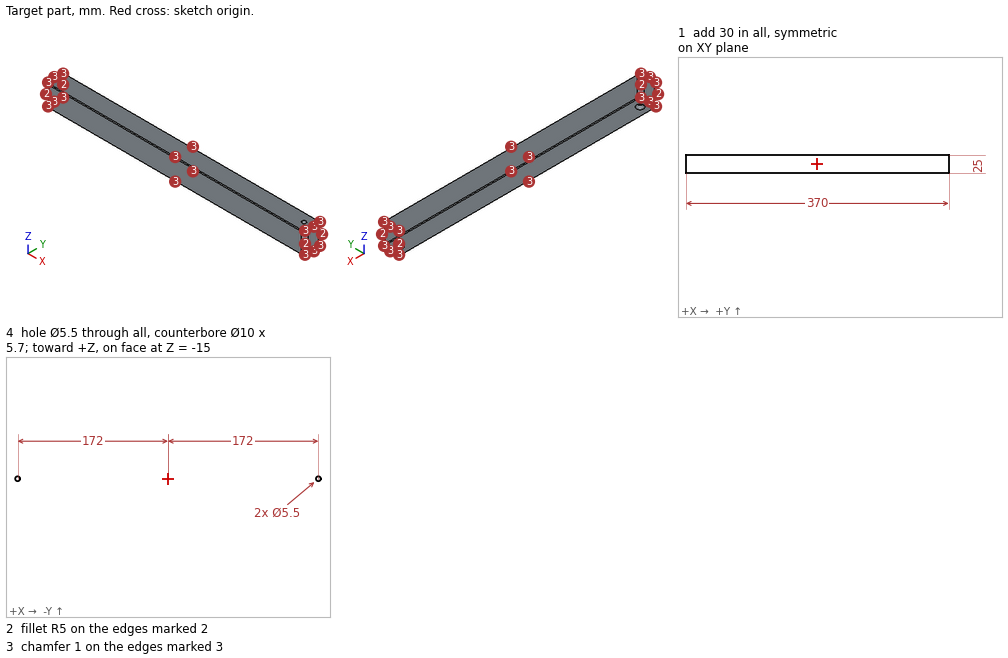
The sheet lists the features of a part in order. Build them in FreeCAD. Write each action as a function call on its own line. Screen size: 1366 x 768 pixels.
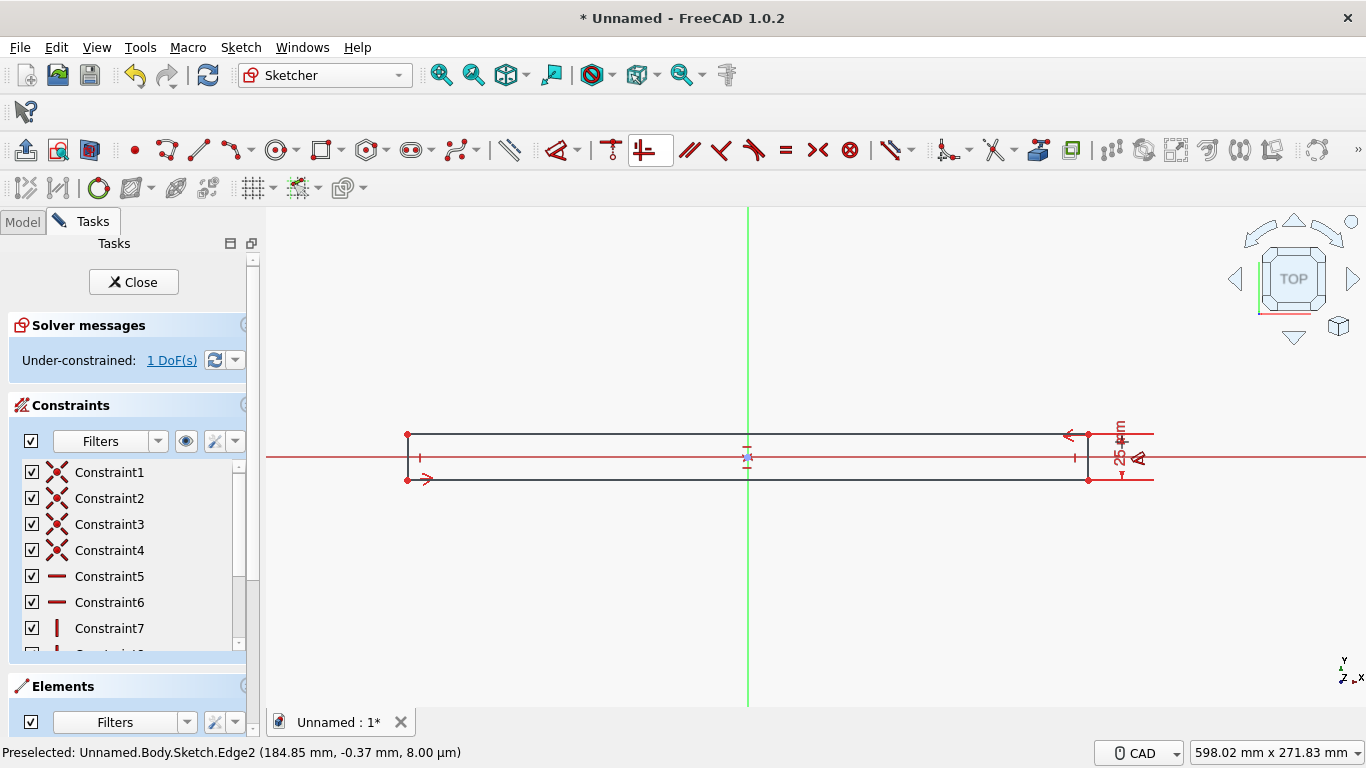
click(612, 480)
click(592, 514)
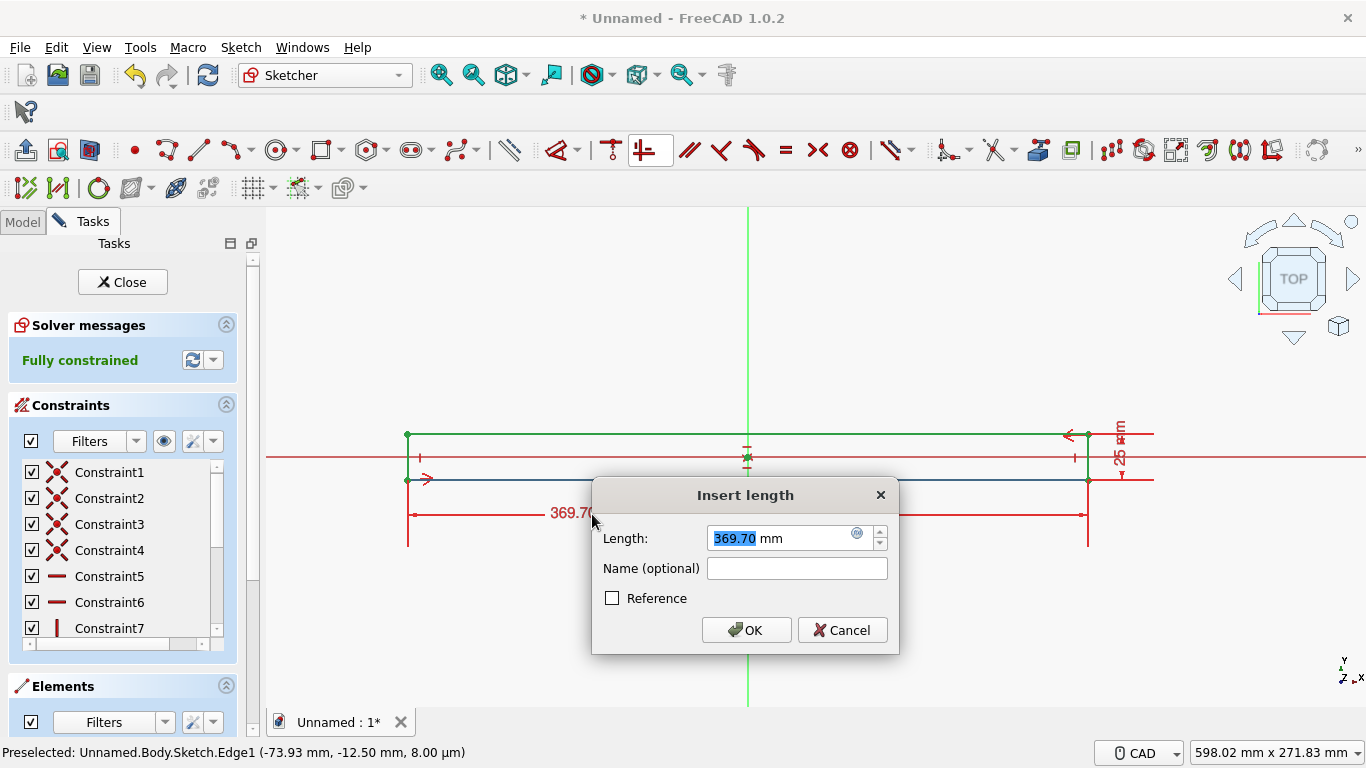
text(370)
key(Return)
key(Escape)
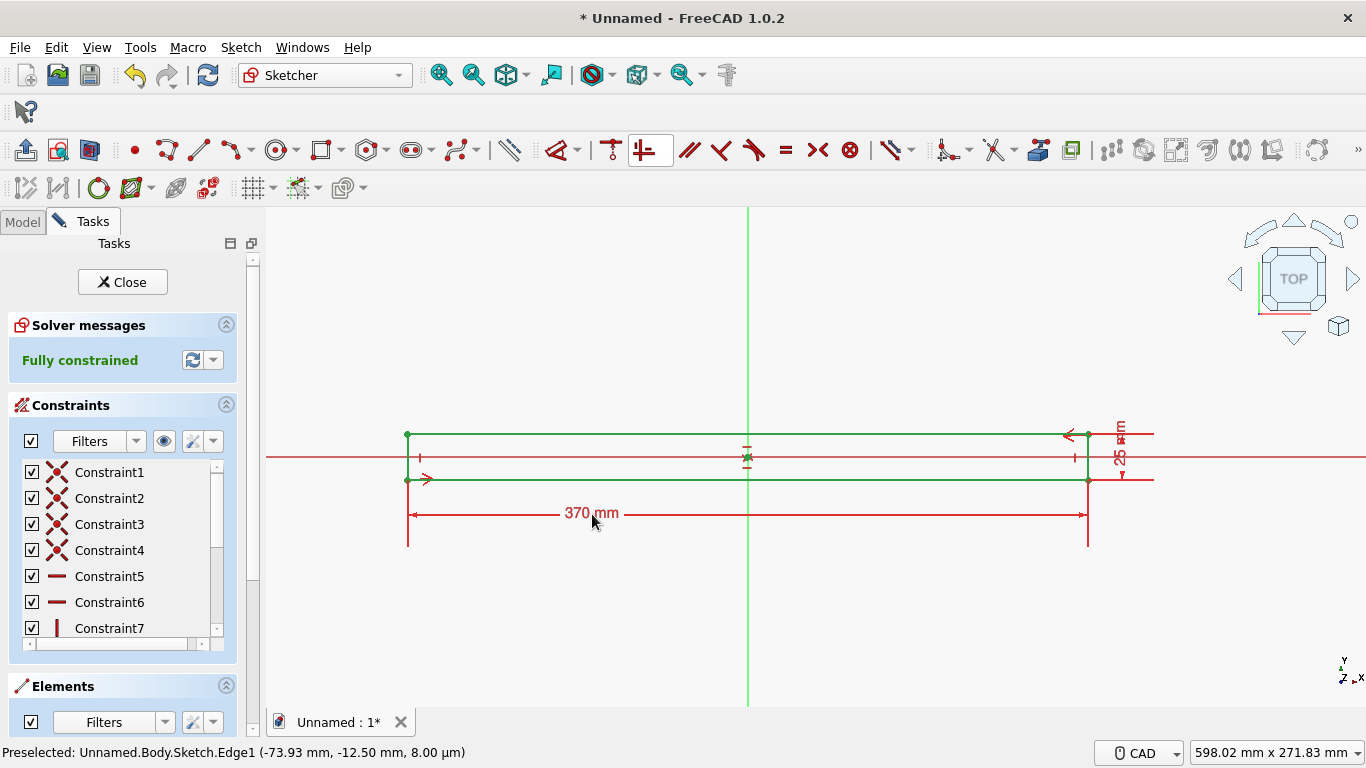
click(123, 282)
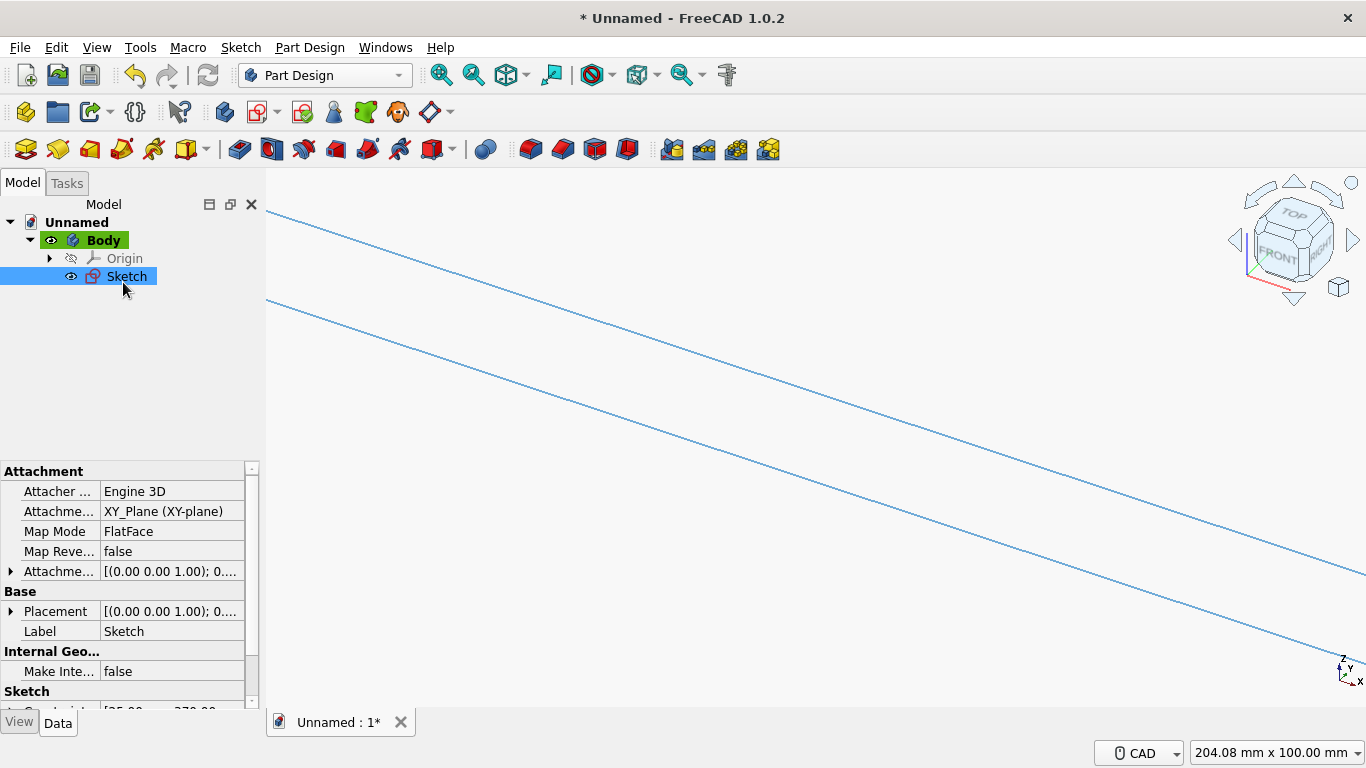
click(26, 150)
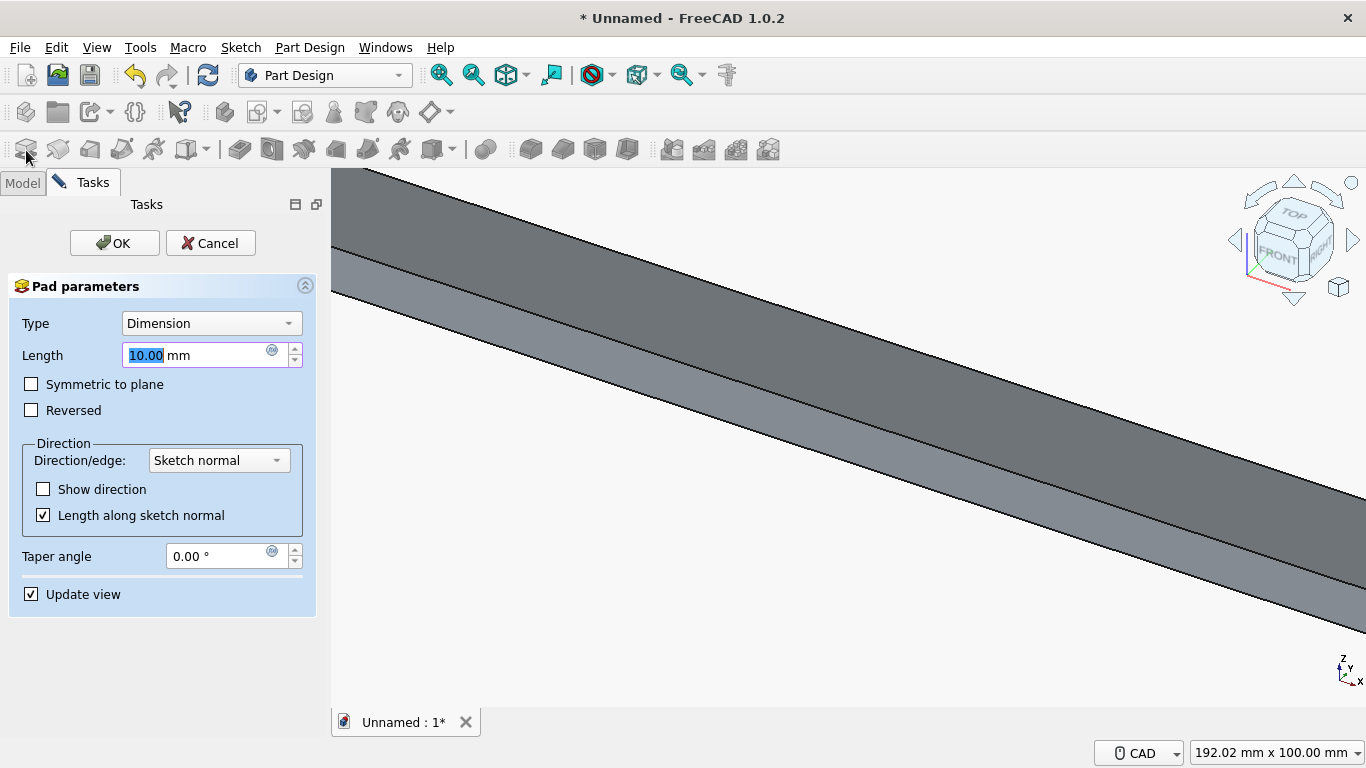
text(30)
key(Tab)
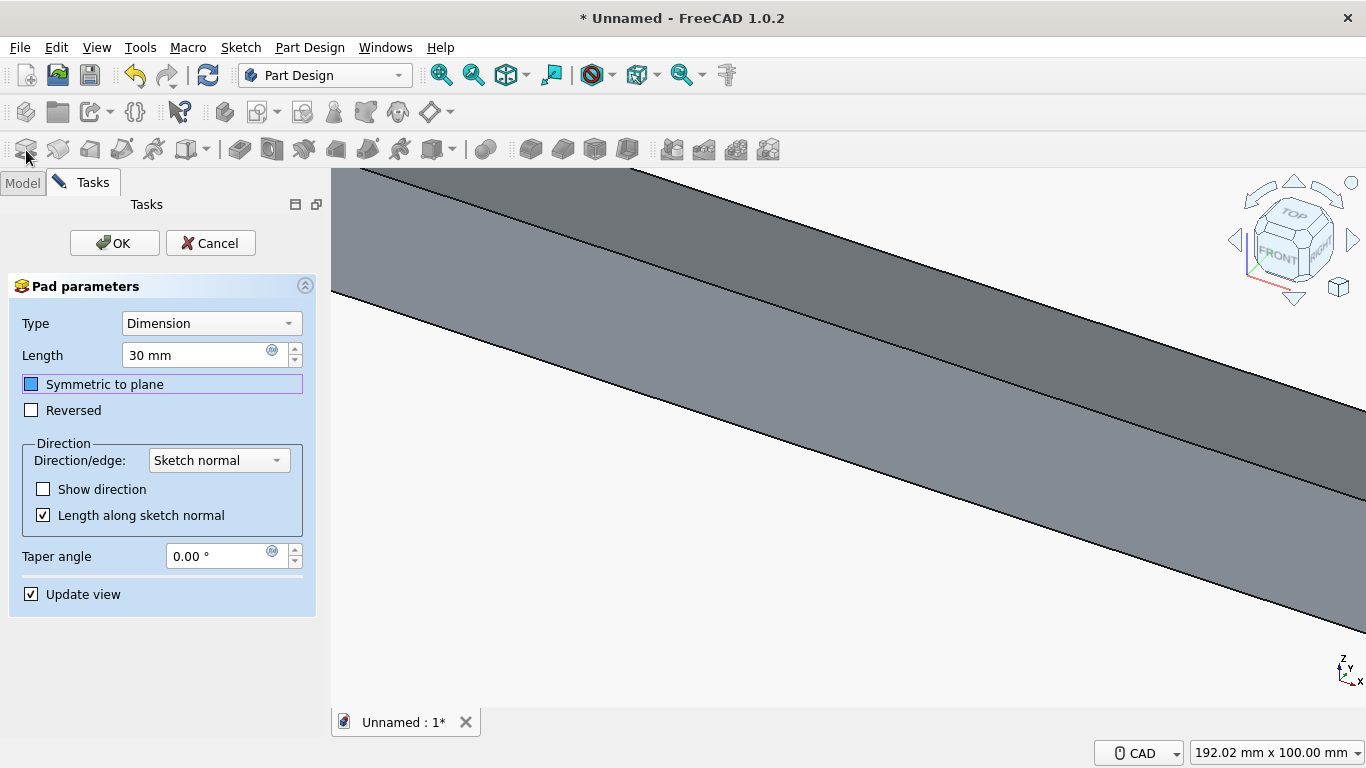
click(30, 384)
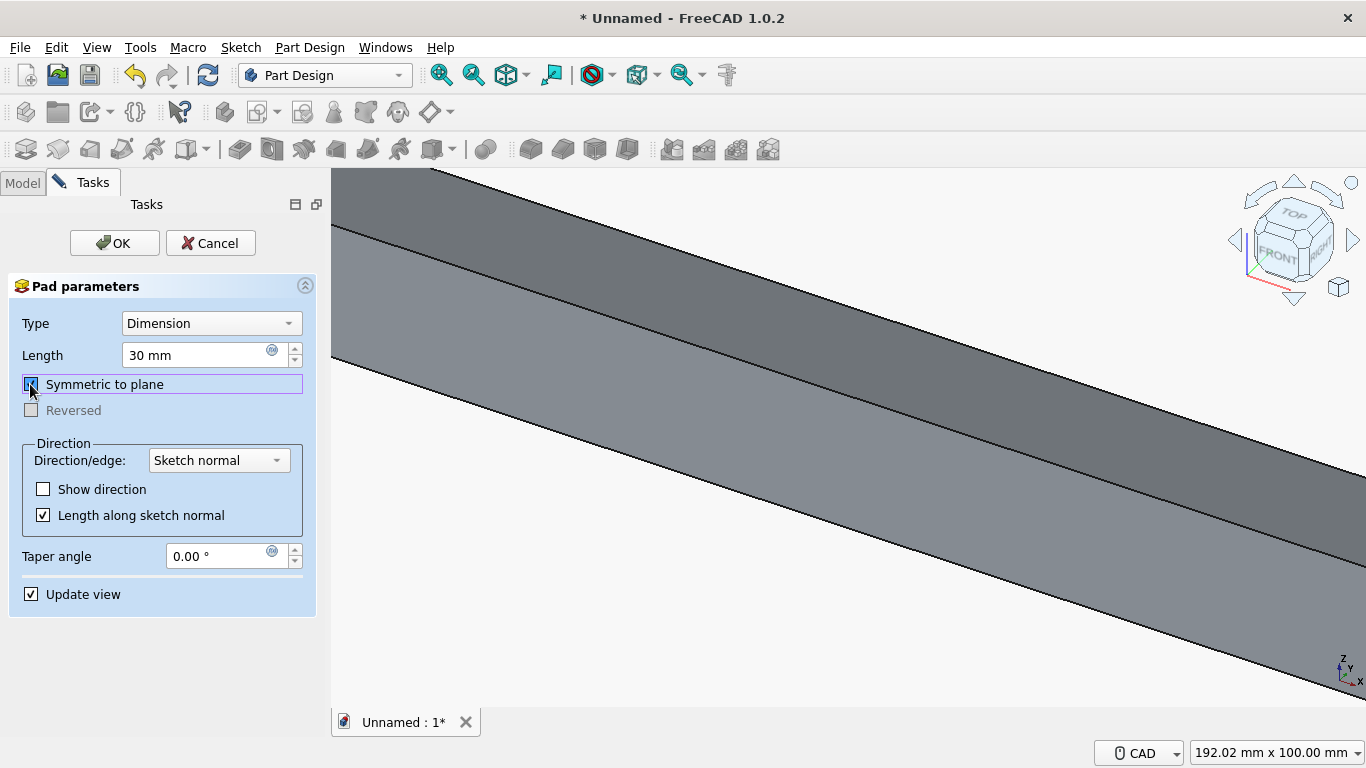
click(115, 243)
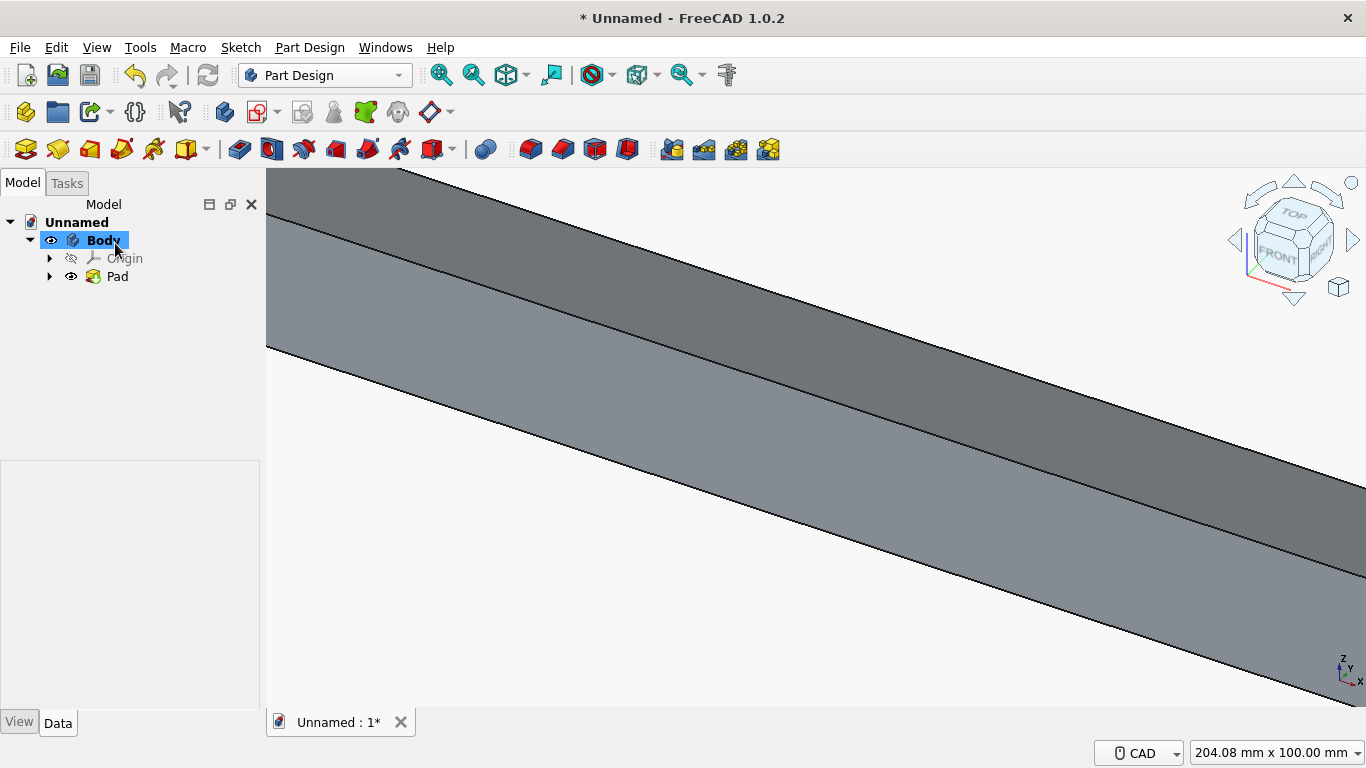
key(v)
key(f)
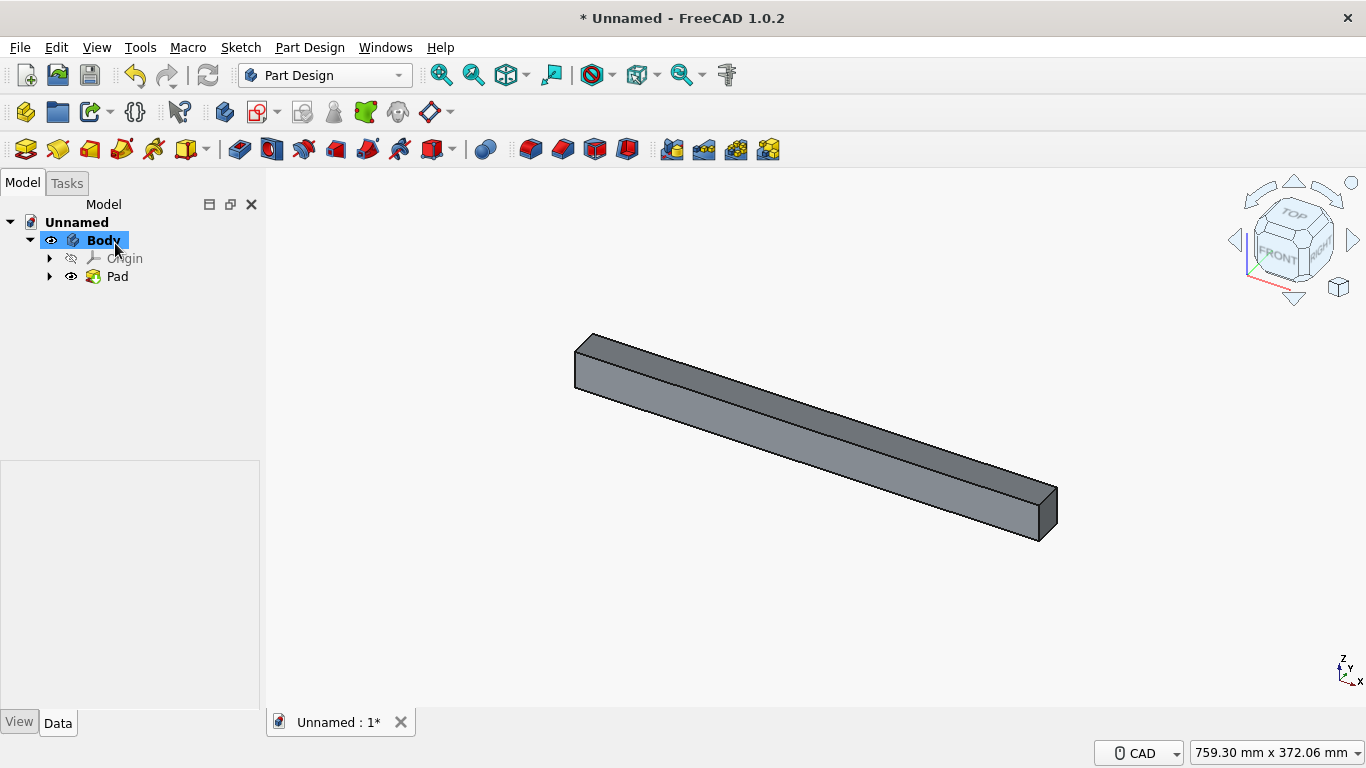
click(1039, 522)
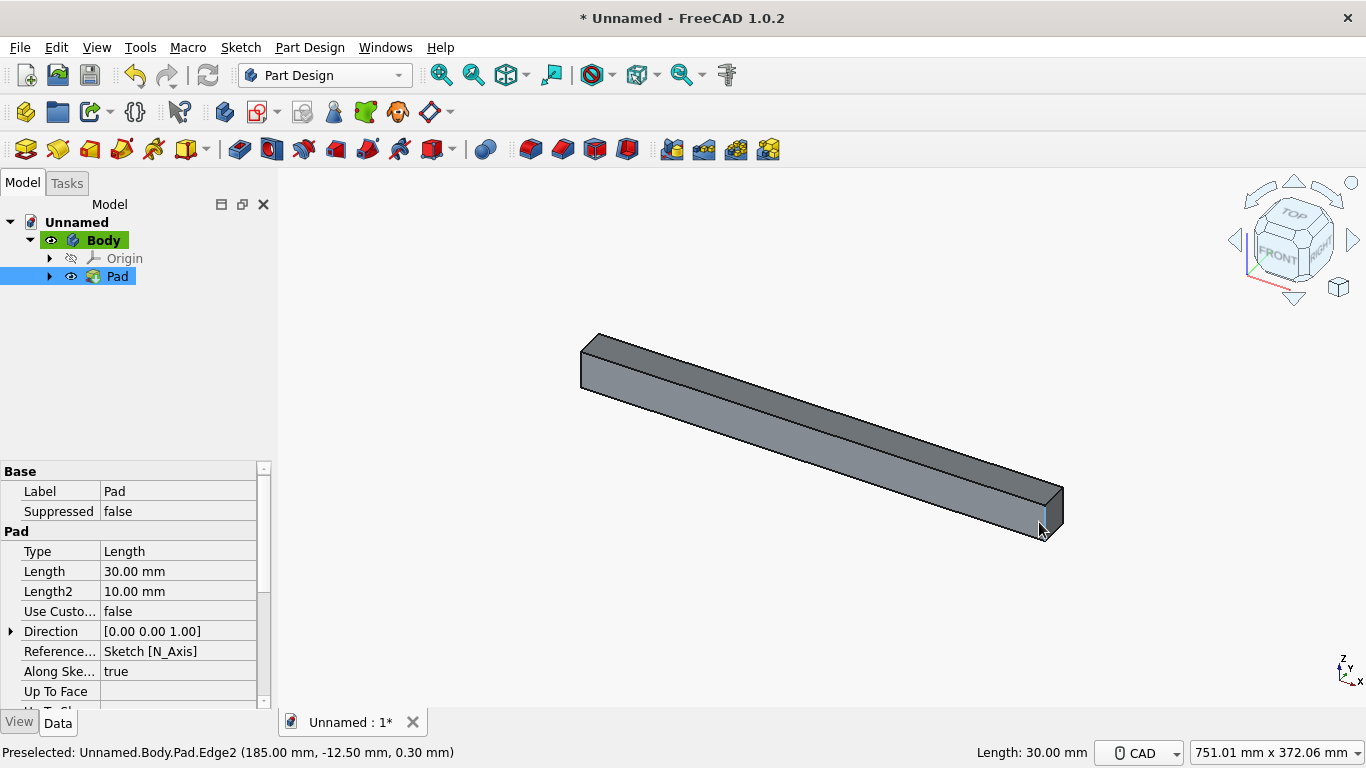
key(0)